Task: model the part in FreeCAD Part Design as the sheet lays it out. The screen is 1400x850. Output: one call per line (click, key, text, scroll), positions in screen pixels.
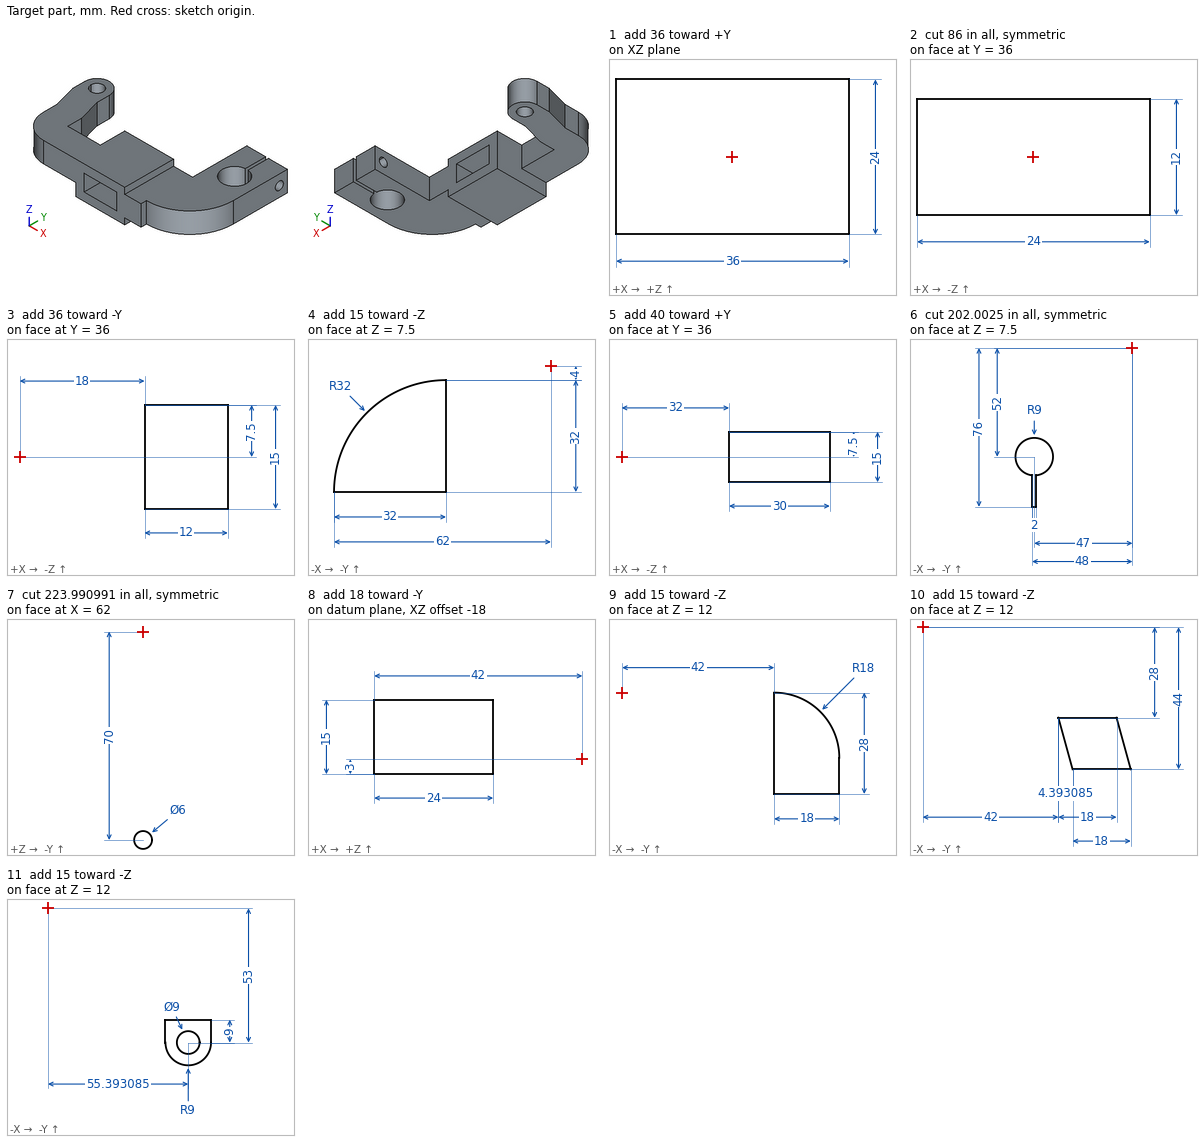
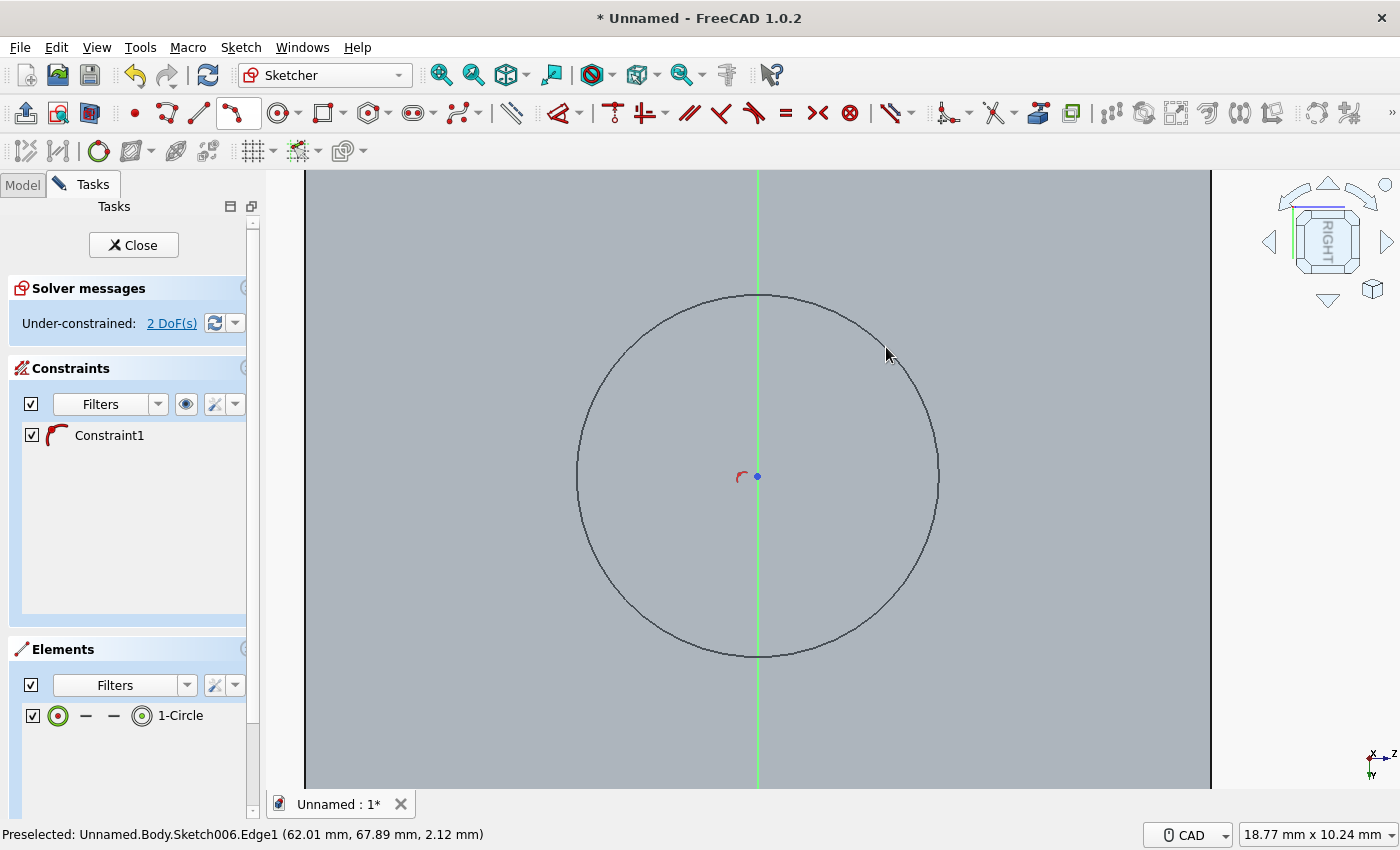
key(d)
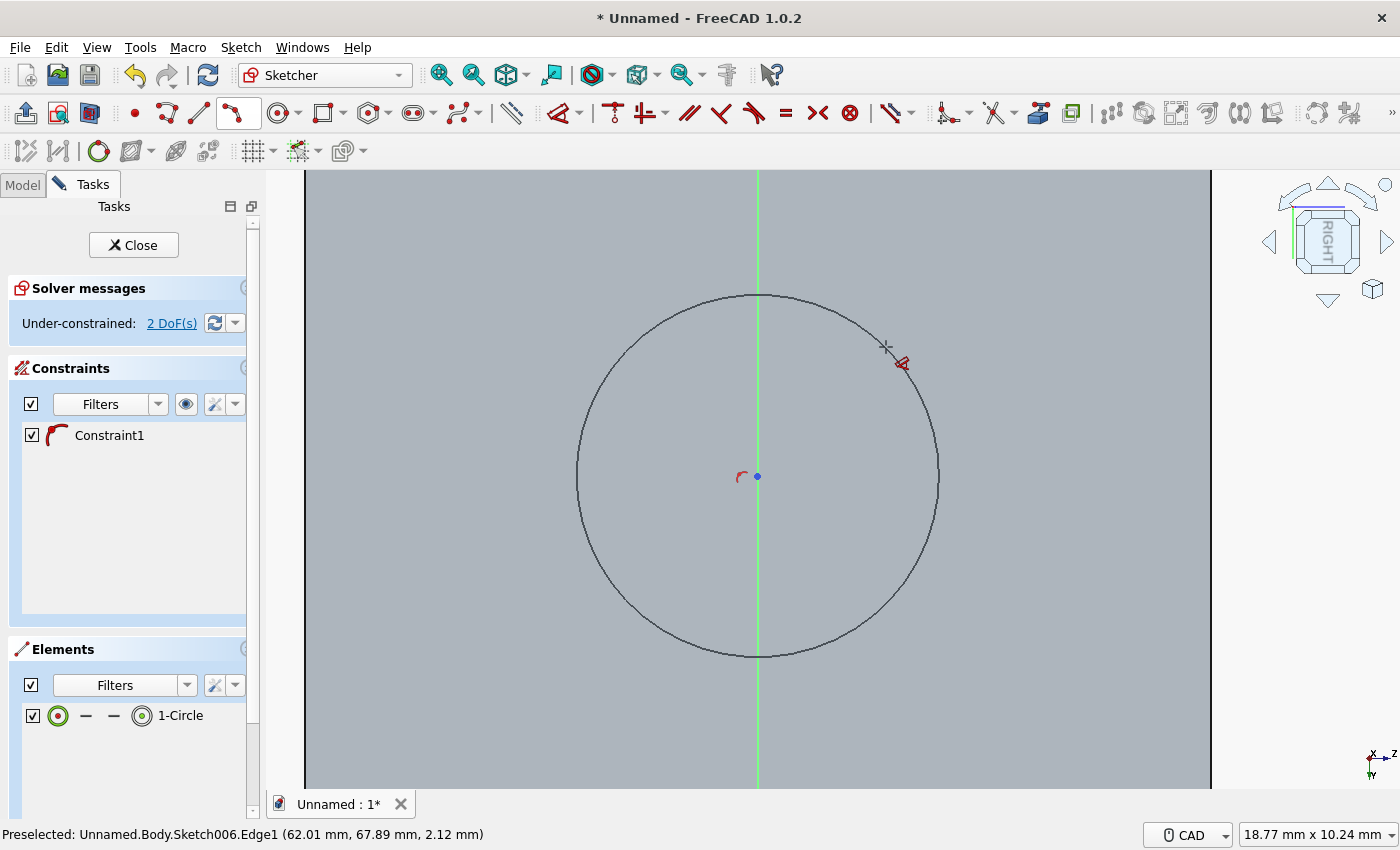
click(885, 347)
click(907, 324)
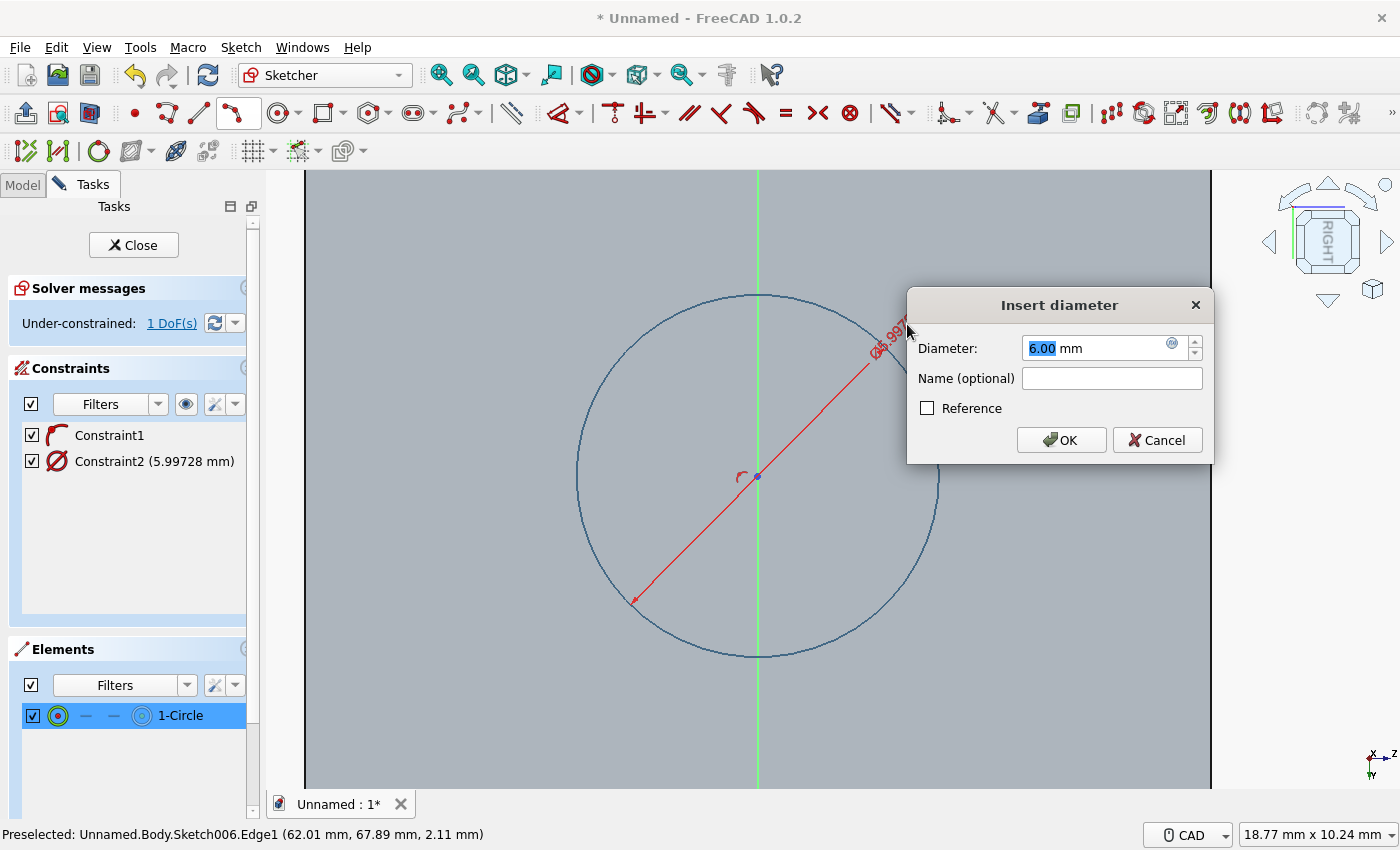
text(6)
key(Return)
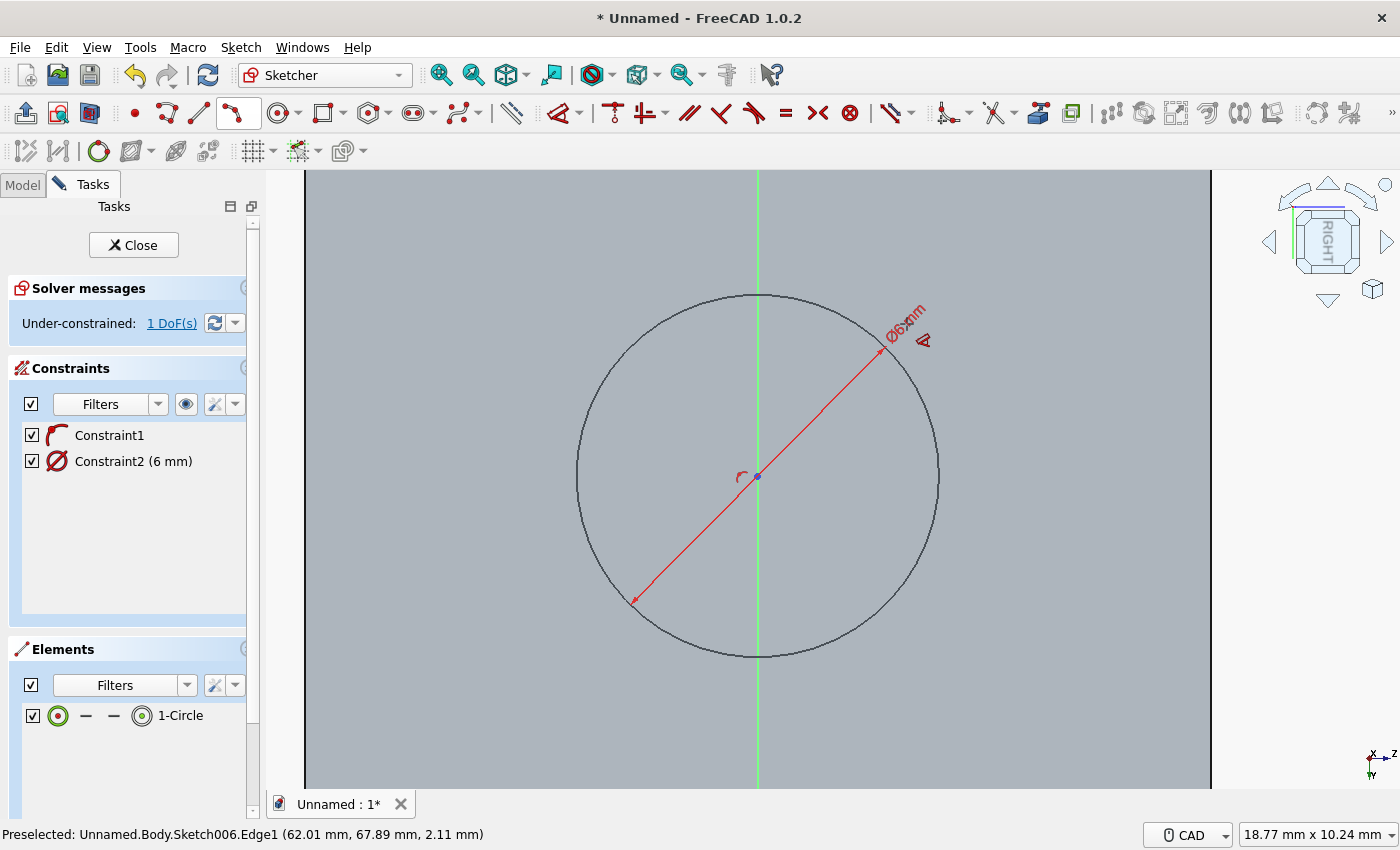
click(758, 476)
click(792, 337)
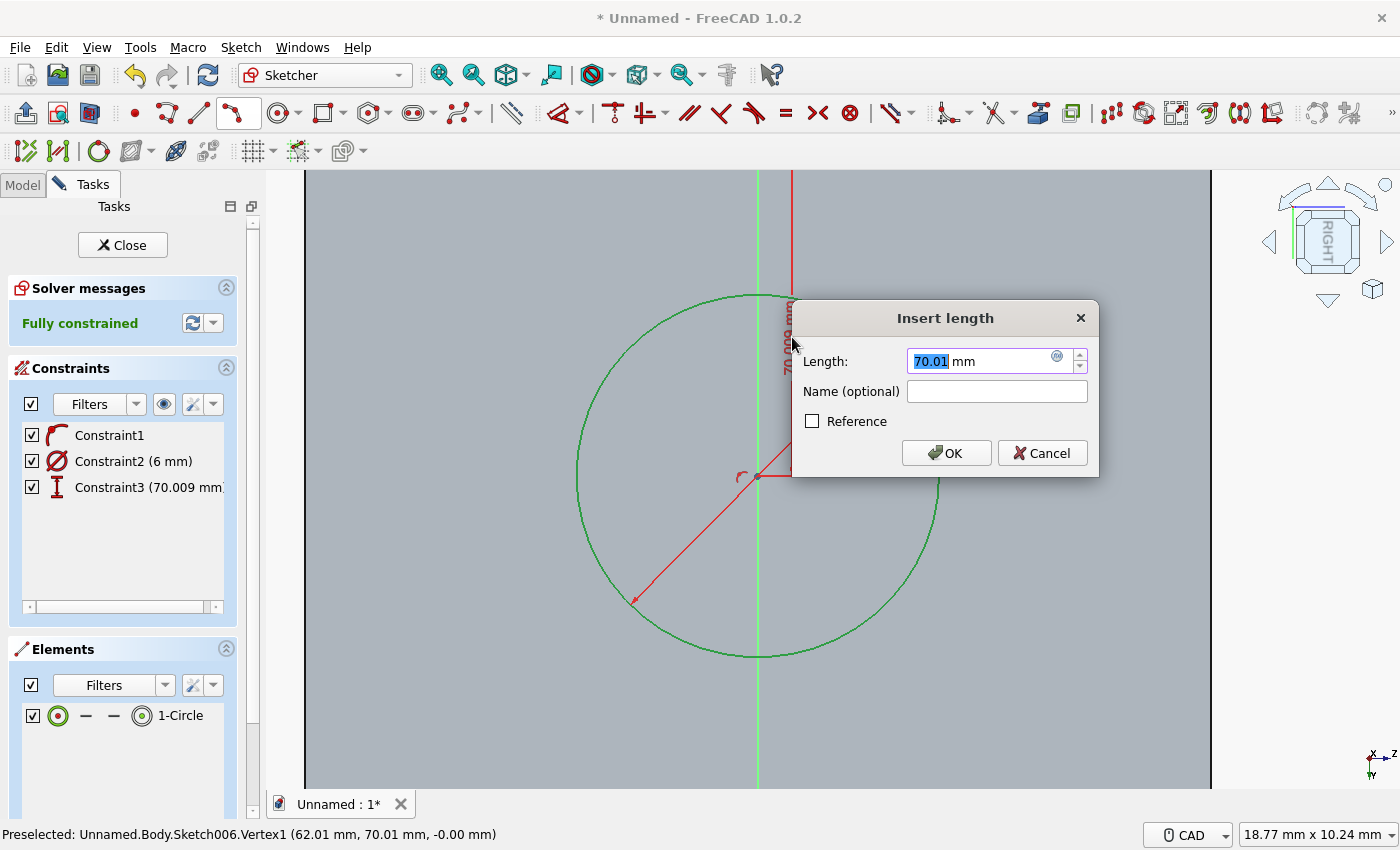
text(70)
key(Return)
key(Escape)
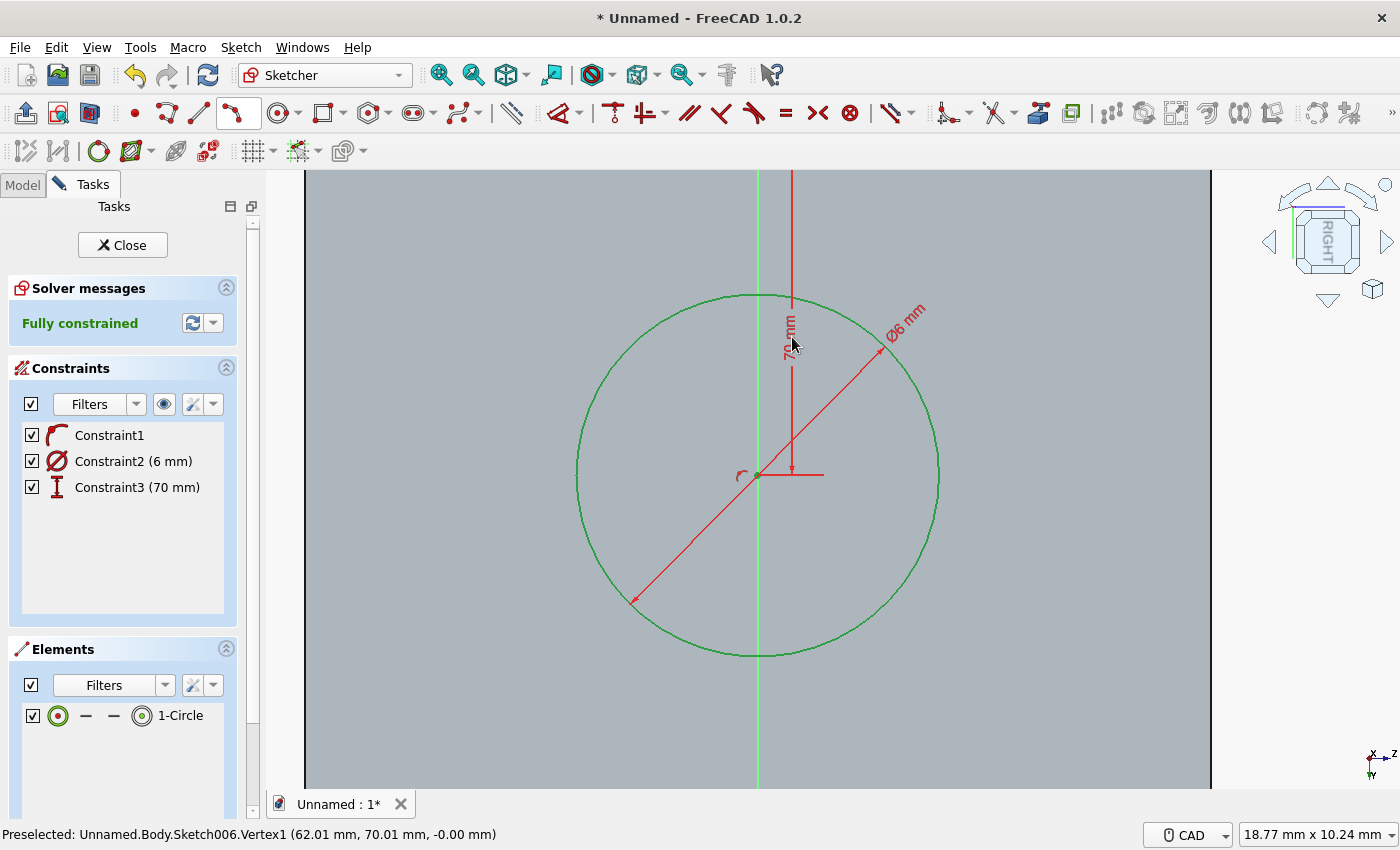
click(123, 245)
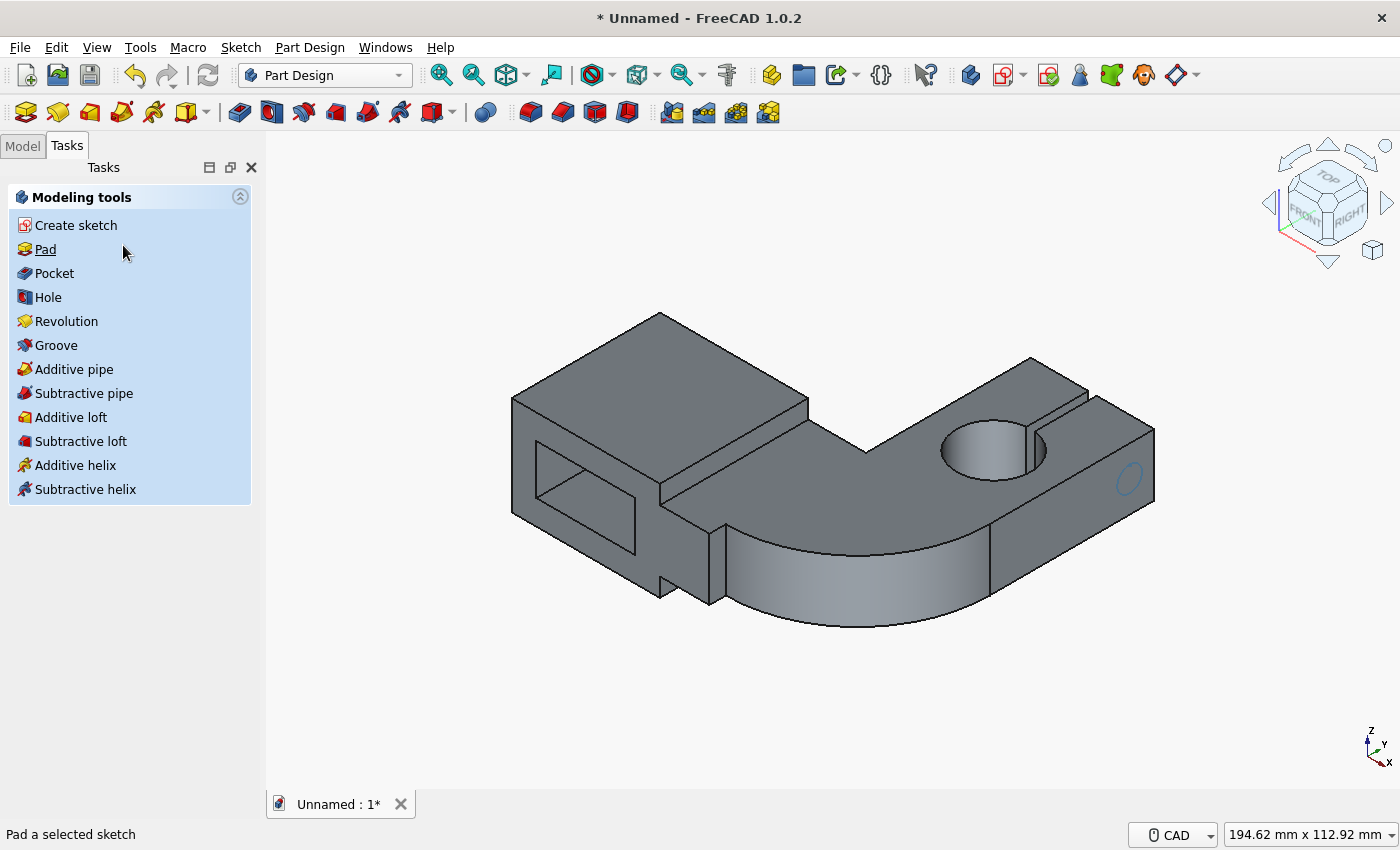
click(240, 112)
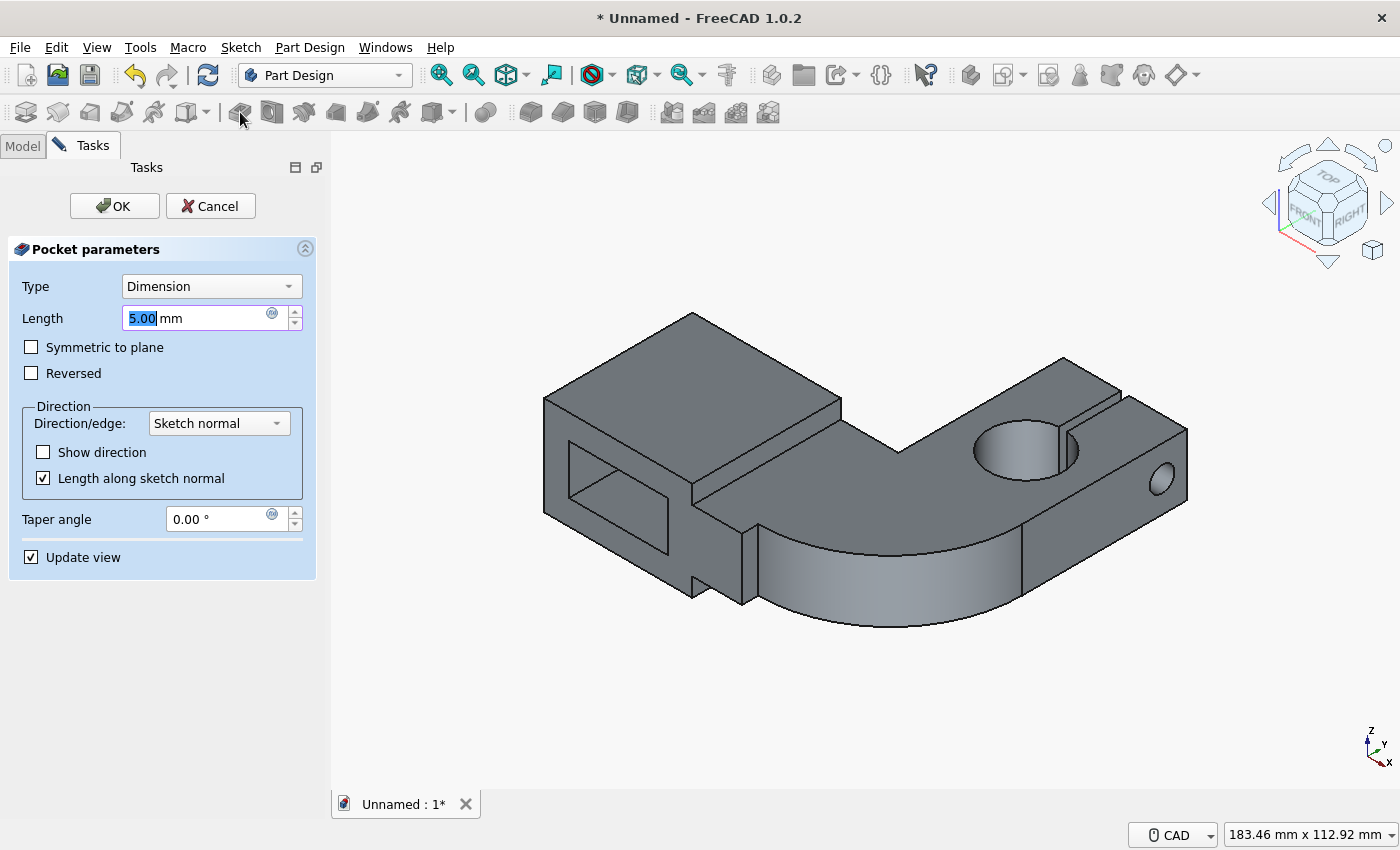
text(223.990991)
key(Tab)